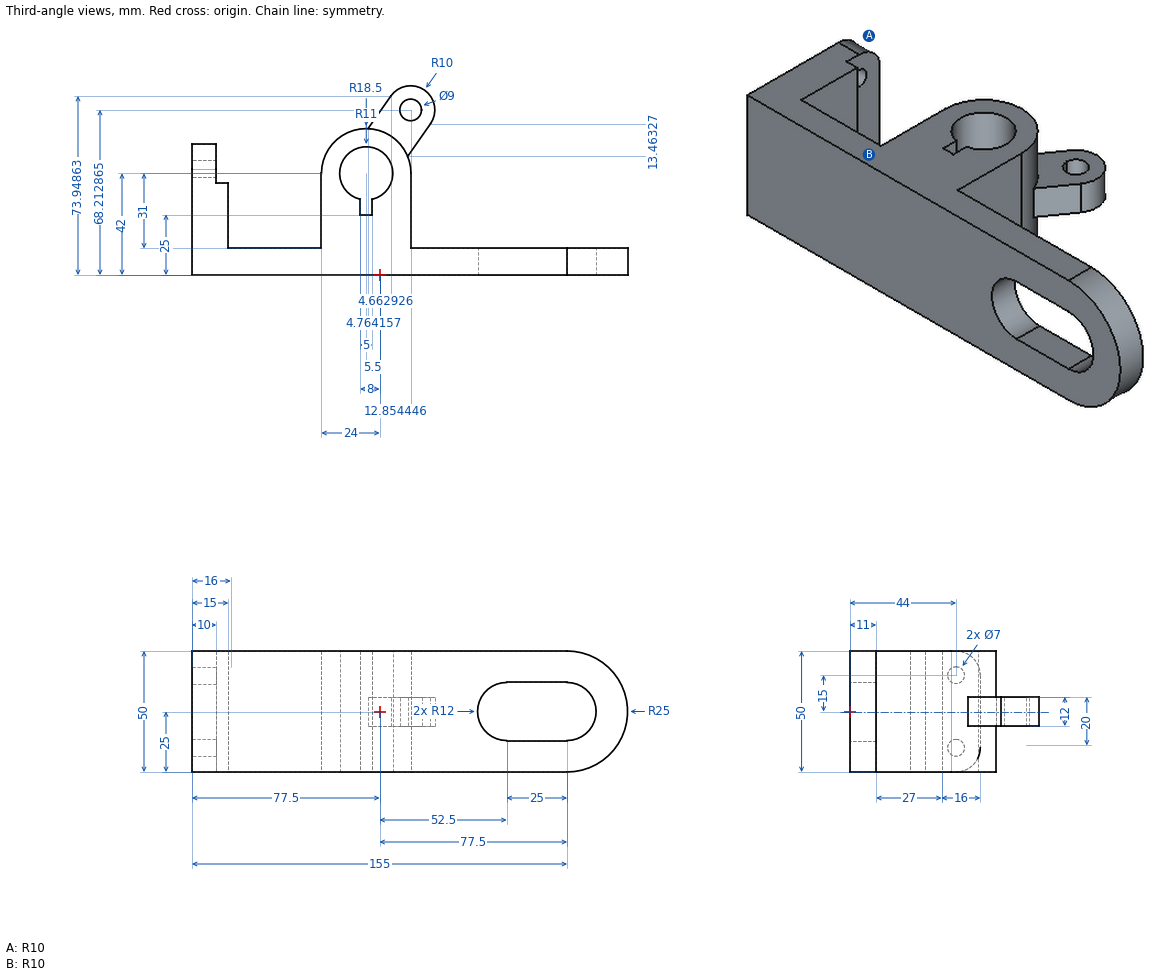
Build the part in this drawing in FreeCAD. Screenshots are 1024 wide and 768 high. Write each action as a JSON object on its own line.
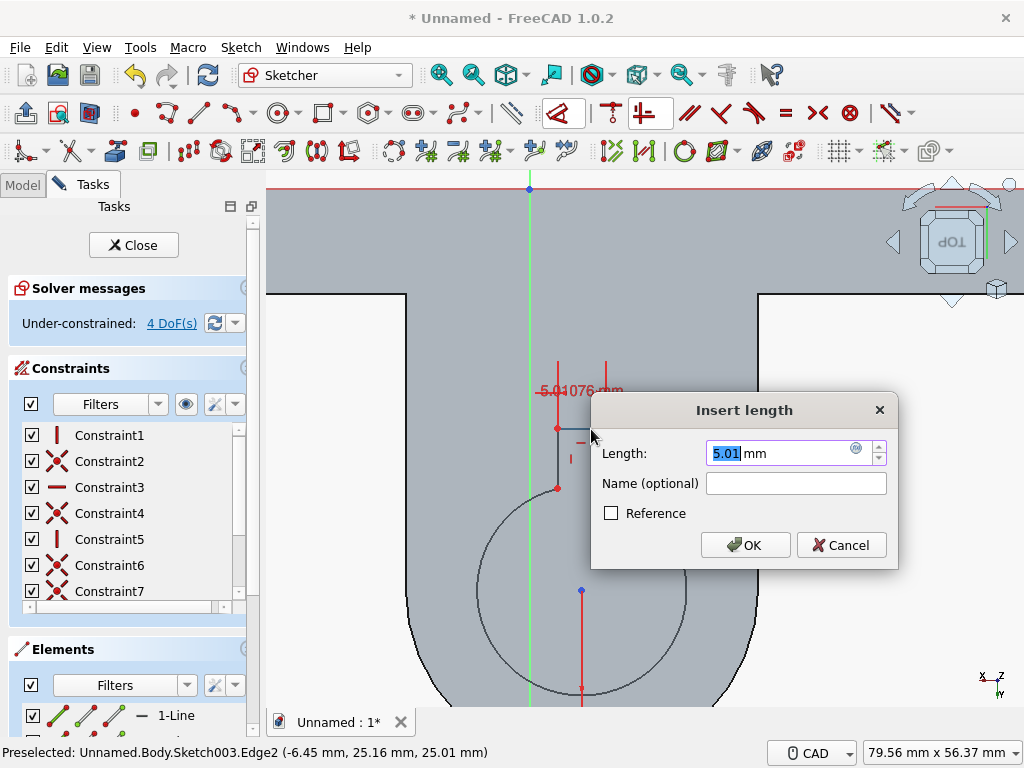
{"action": "type", "text": "5"}
{"action": "key", "text": "Return"}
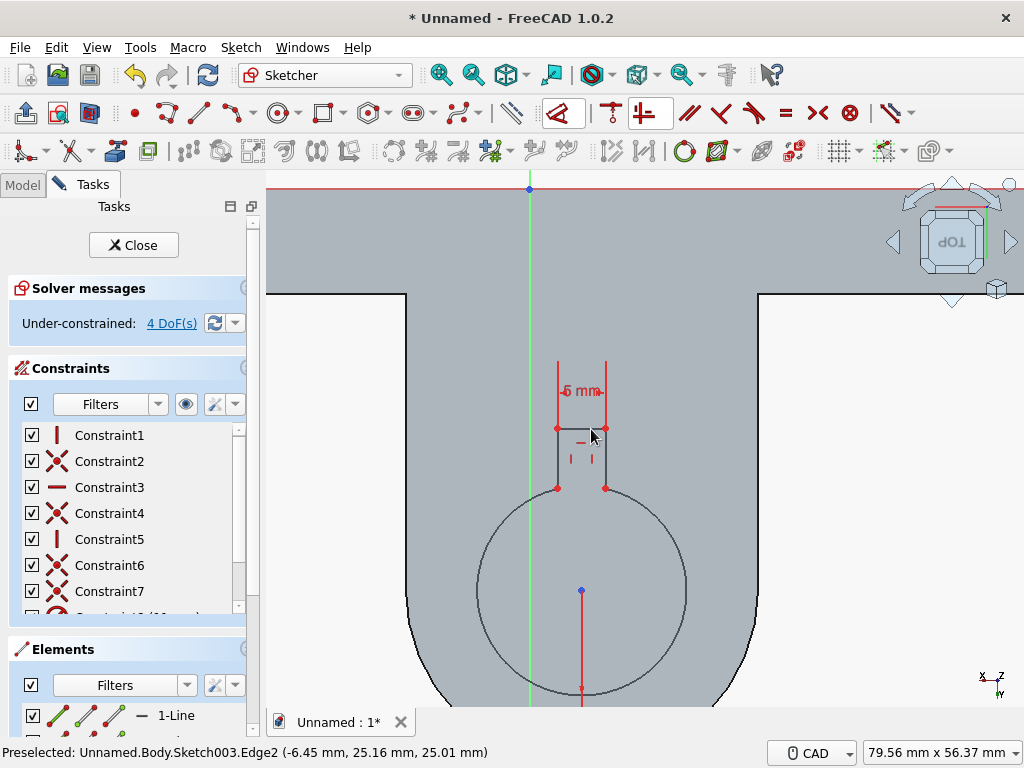
{"action": "left_click", "coordinate": [606, 489]}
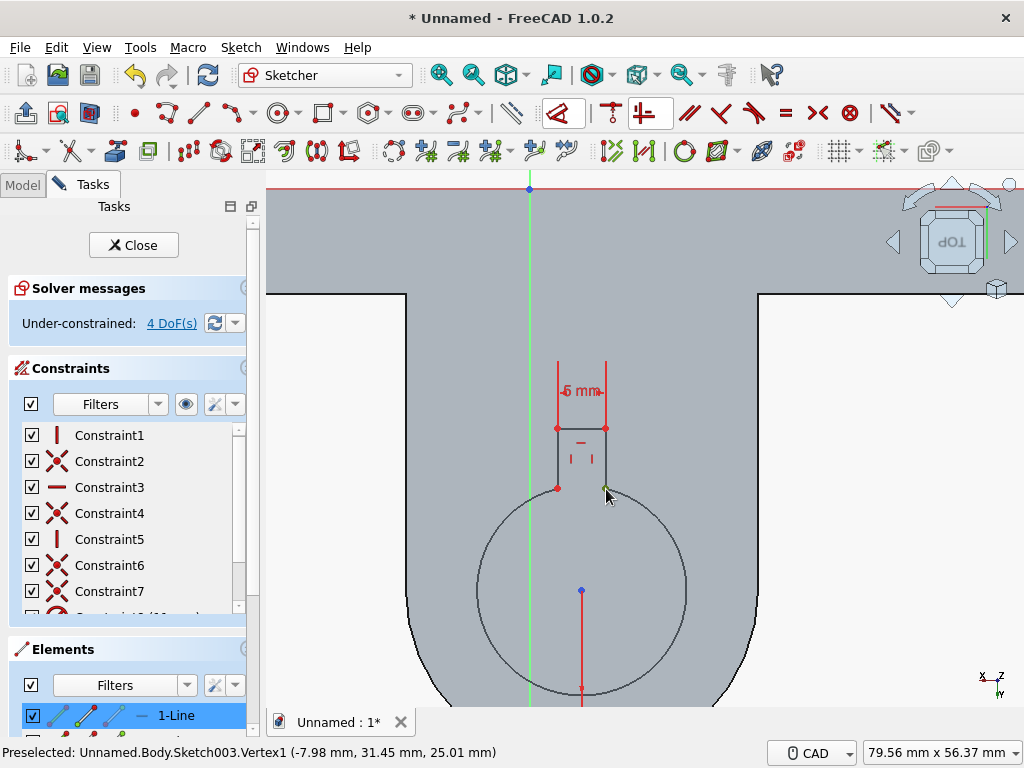
{"action": "left_click", "coordinate": [580, 114]}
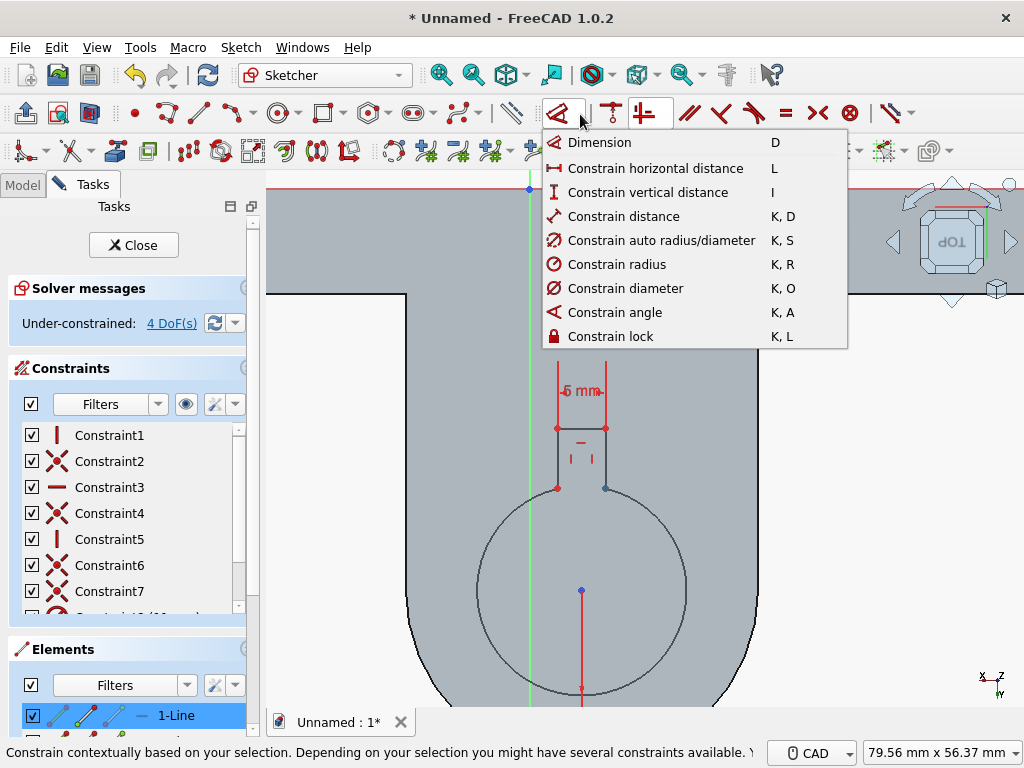
{"action": "left_click", "coordinate": [695, 168]}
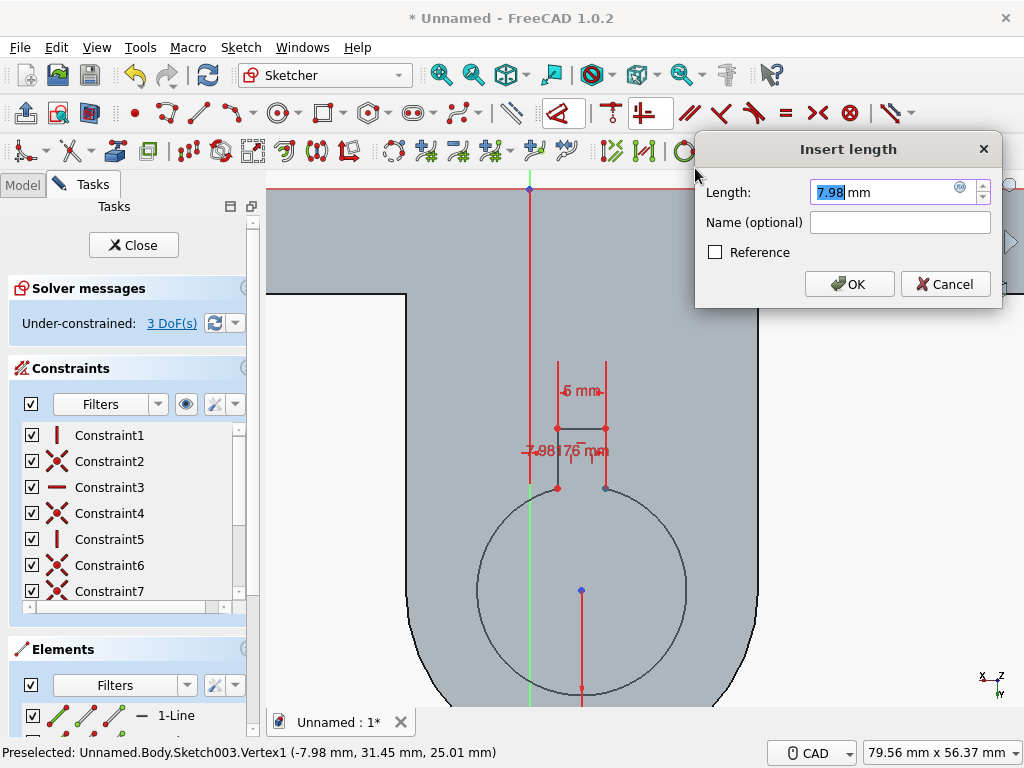
{"action": "type", "text": "8"}
{"action": "key", "text": "Return"}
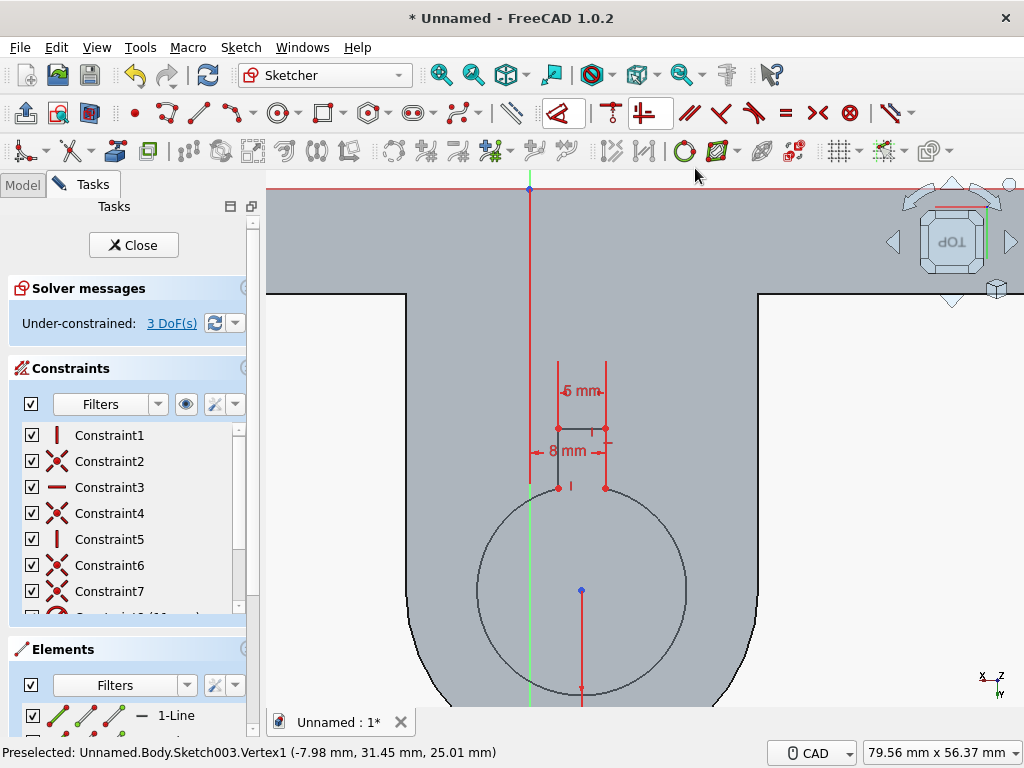
{"action": "left_click", "coordinate": [606, 429]}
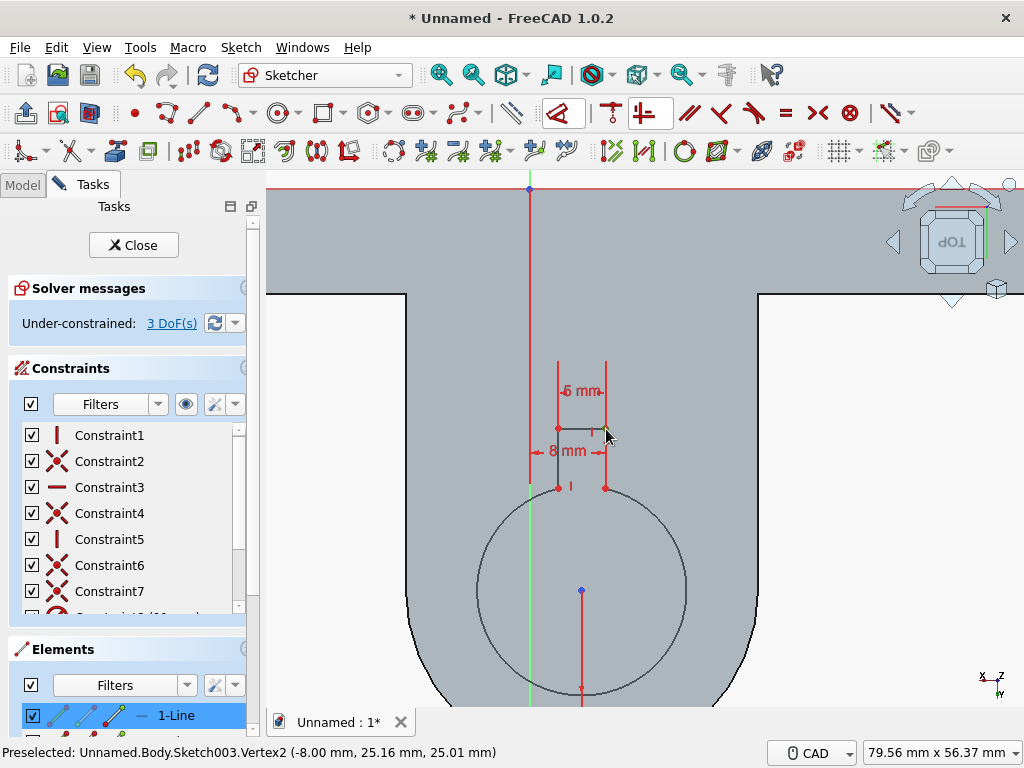
{"action": "key", "text": "i"}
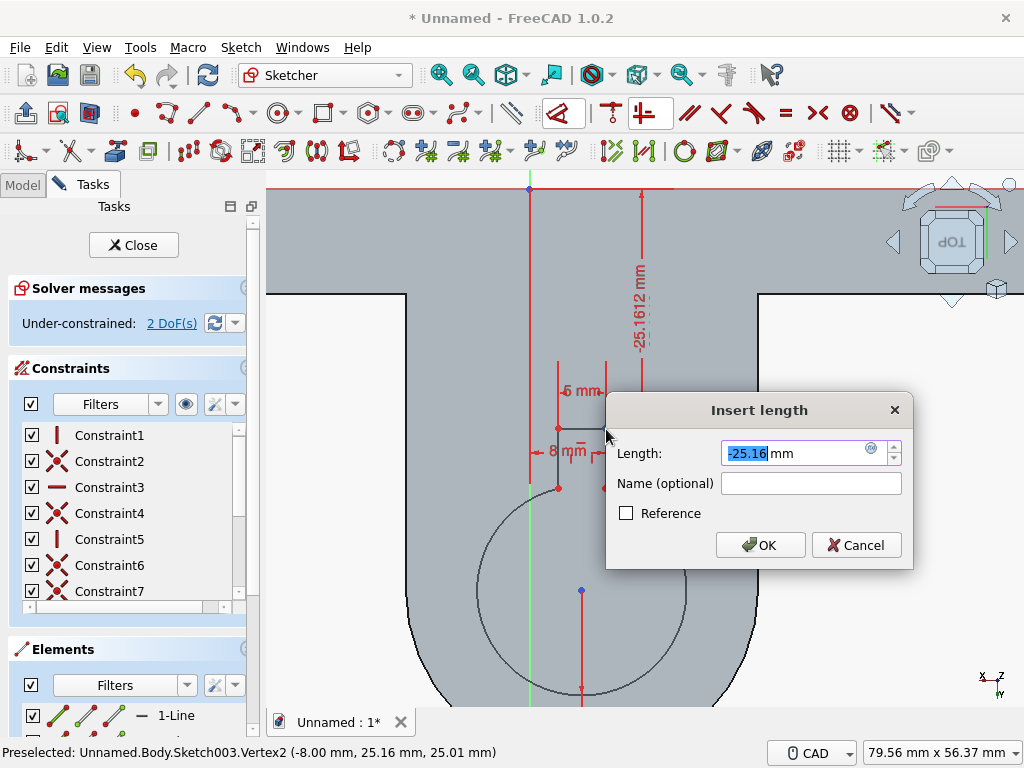
{"action": "type", "text": "-25"}
{"action": "key", "text": "Return"}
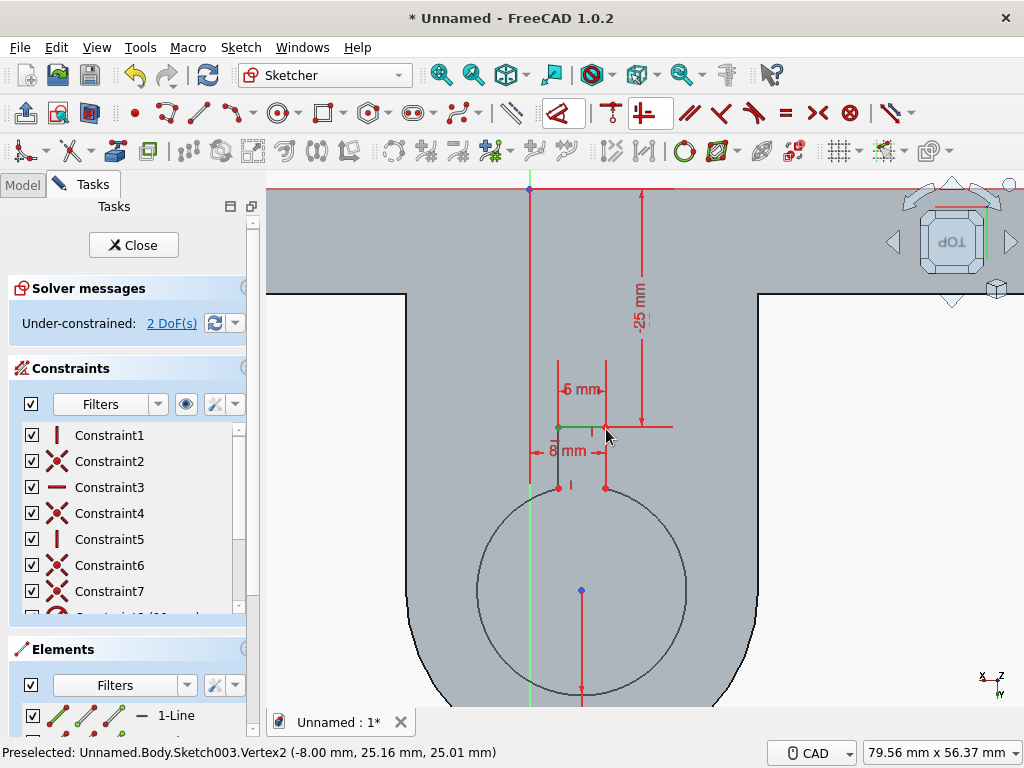
{"action": "left_click", "coordinate": [582, 591]}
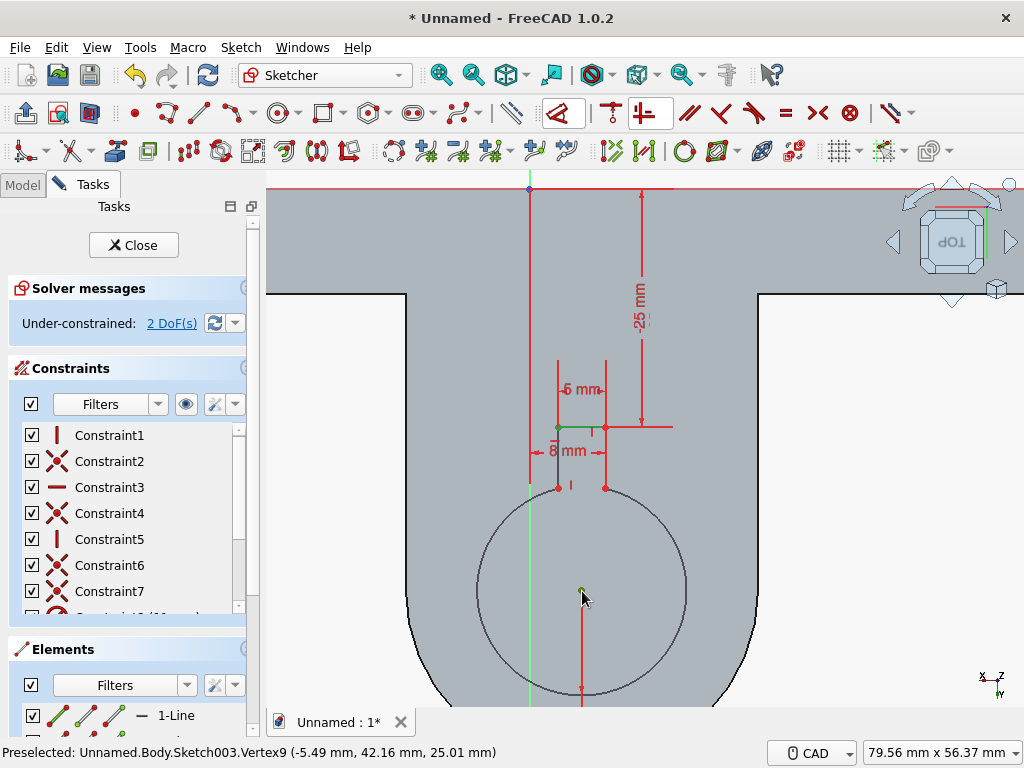
{"action": "left_click", "coordinate": [580, 114]}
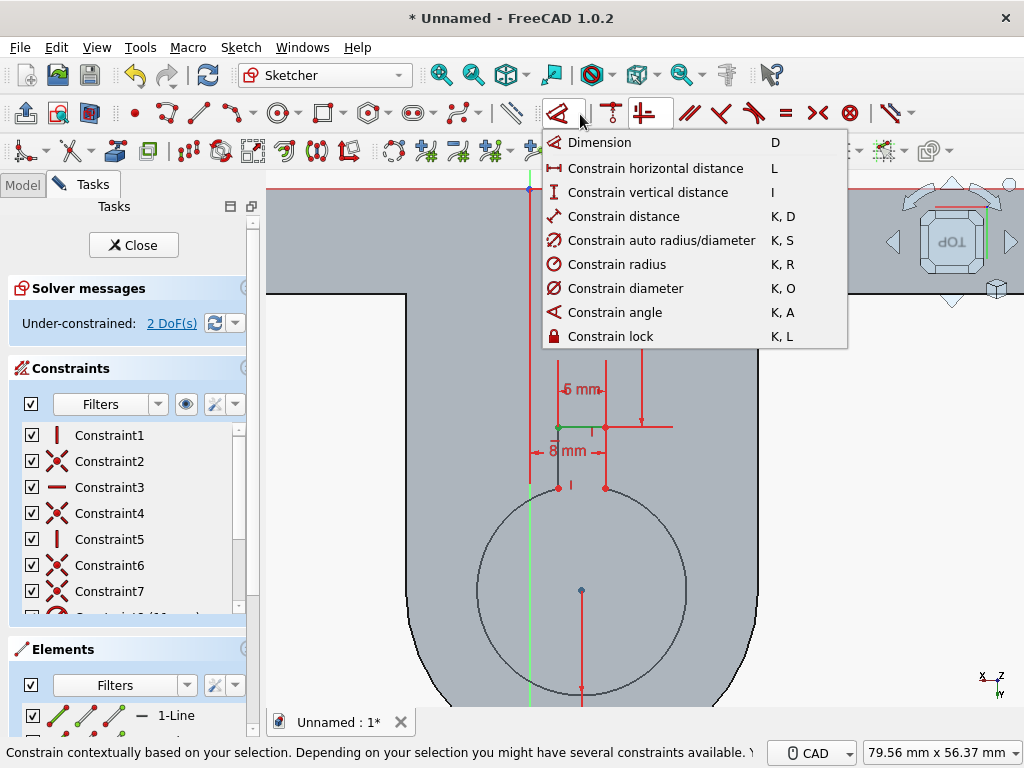
{"action": "left_click", "coordinate": [695, 192]}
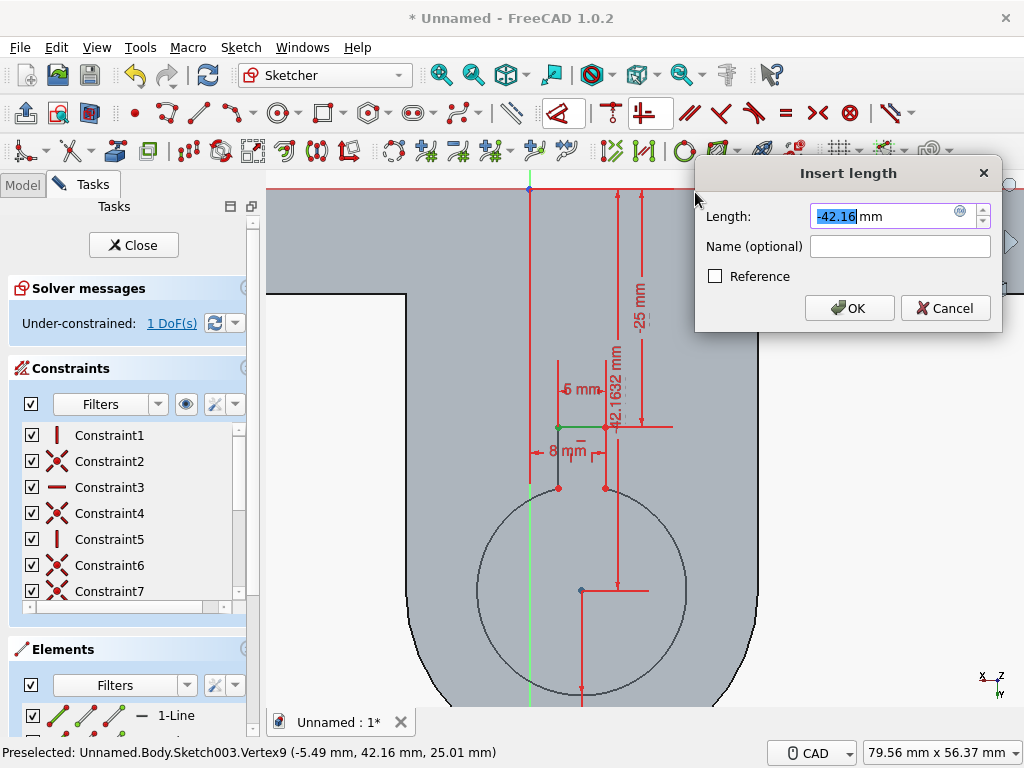
{"action": "type", "text": "-42"}
{"action": "key", "text": "Return"}